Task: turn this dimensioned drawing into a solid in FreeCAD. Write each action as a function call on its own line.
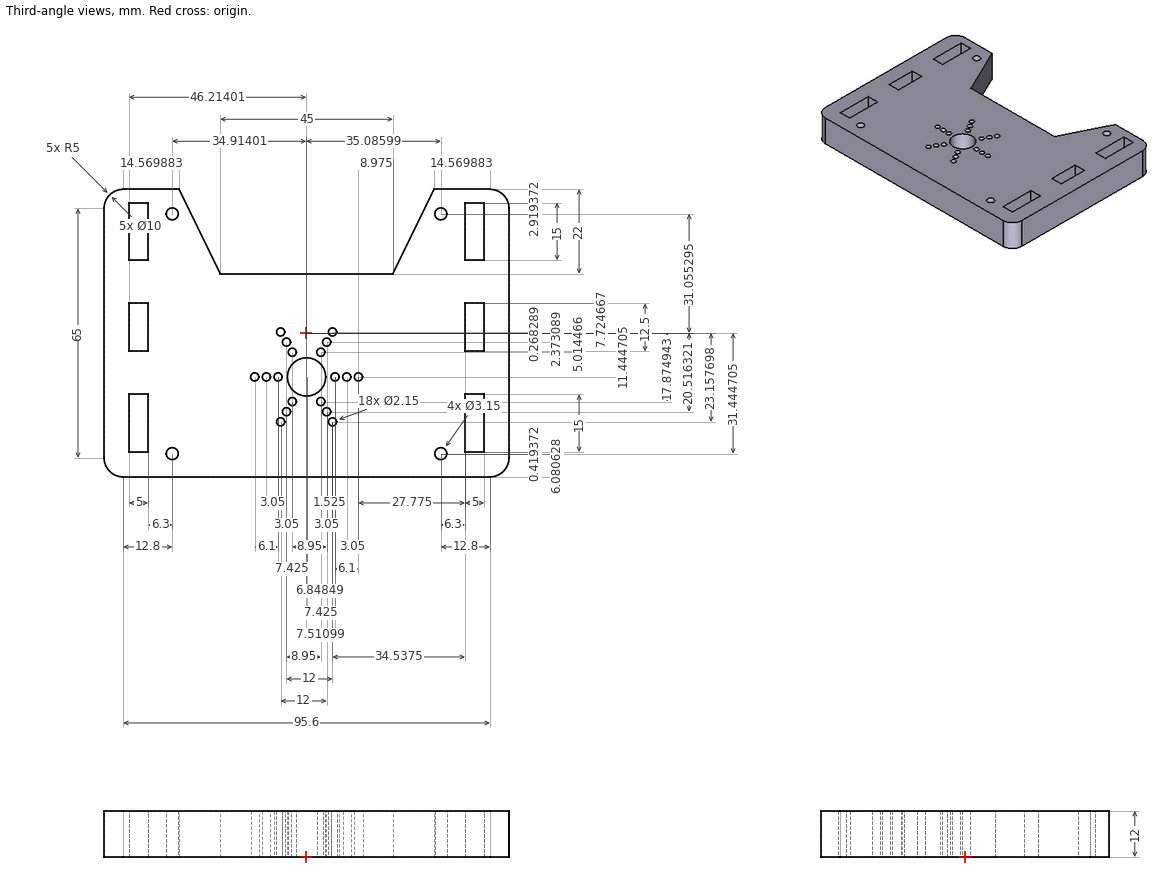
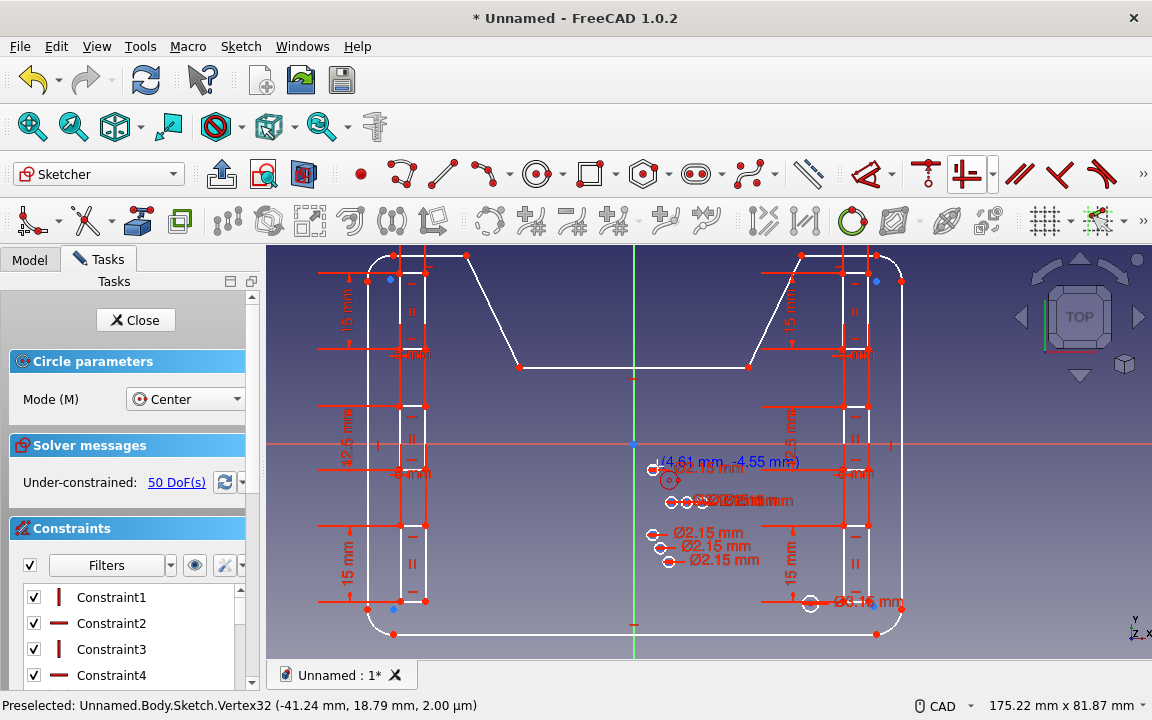
scroll(668, 443, up, 13)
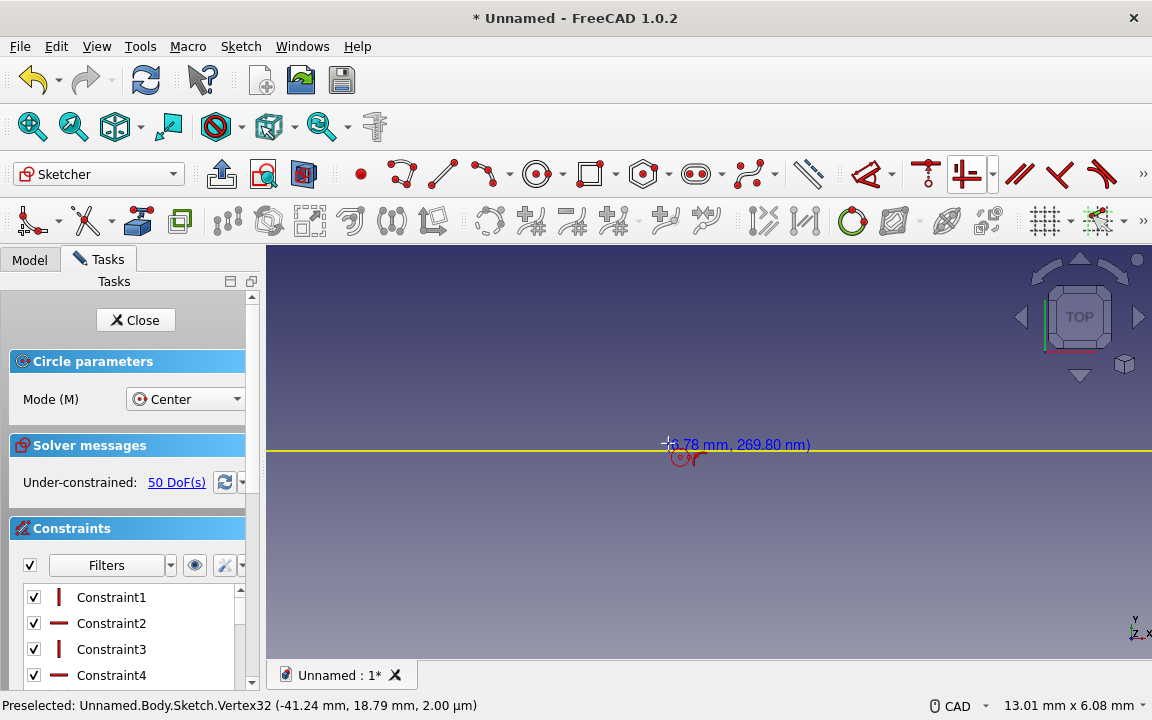
click(667, 432)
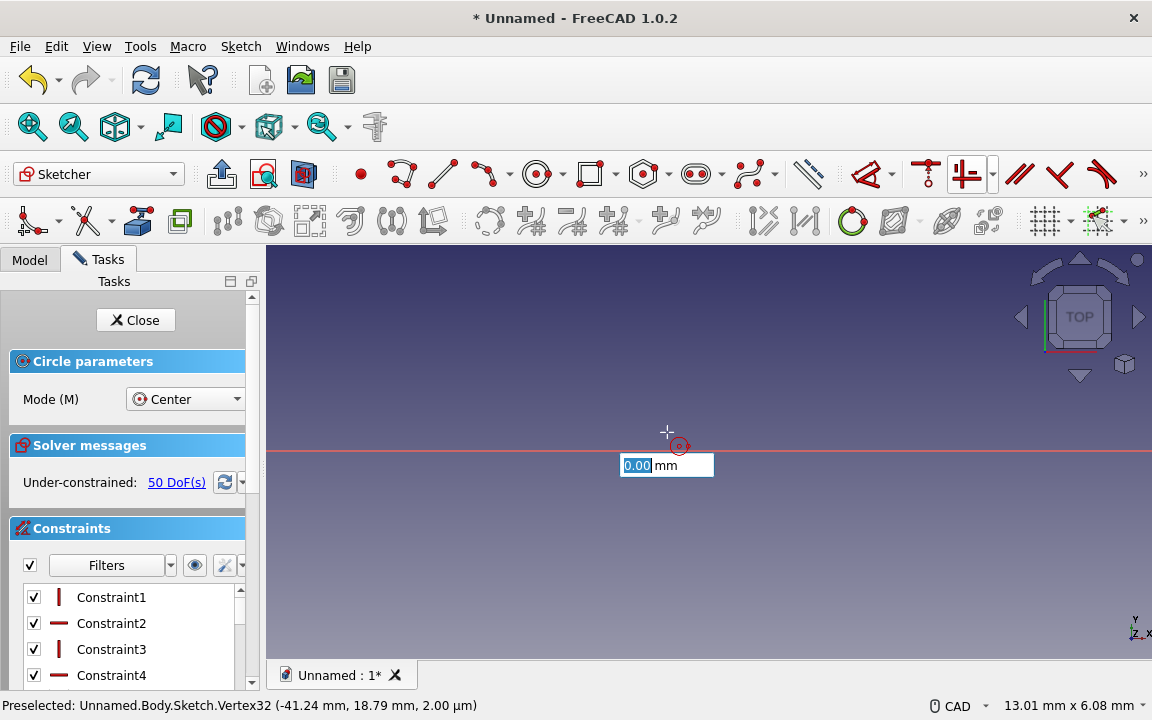
scroll(663, 452, down, 15)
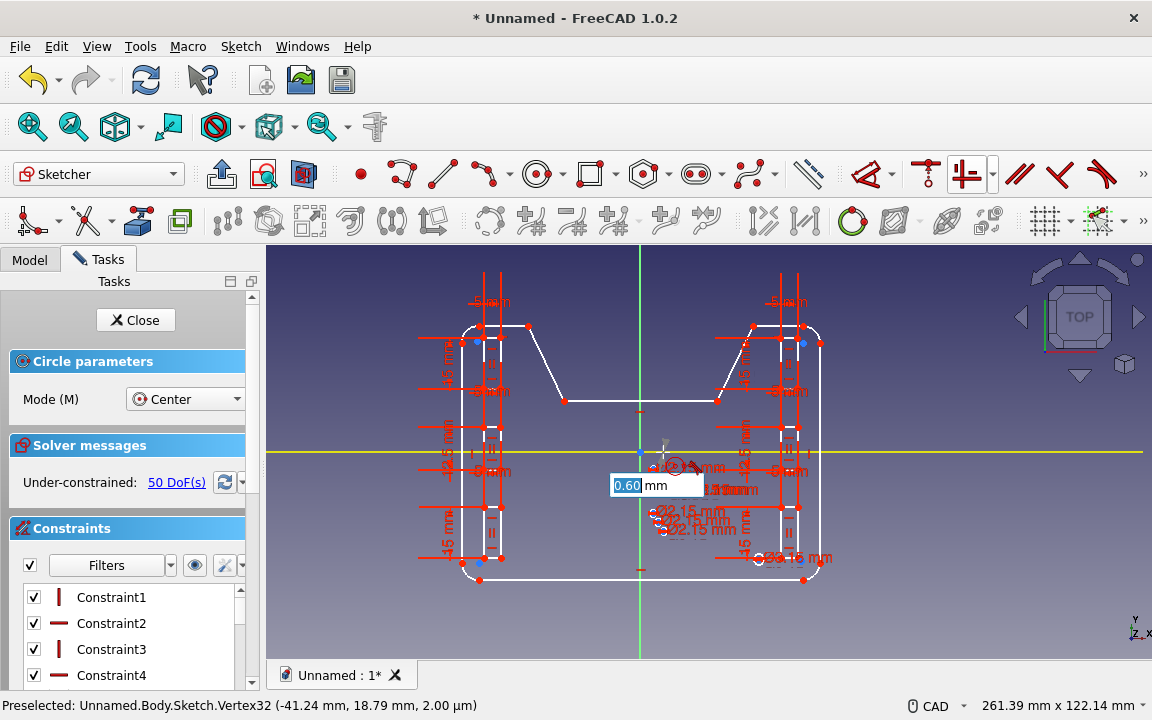
scroll(666, 449, up, 8)
move(665, 447)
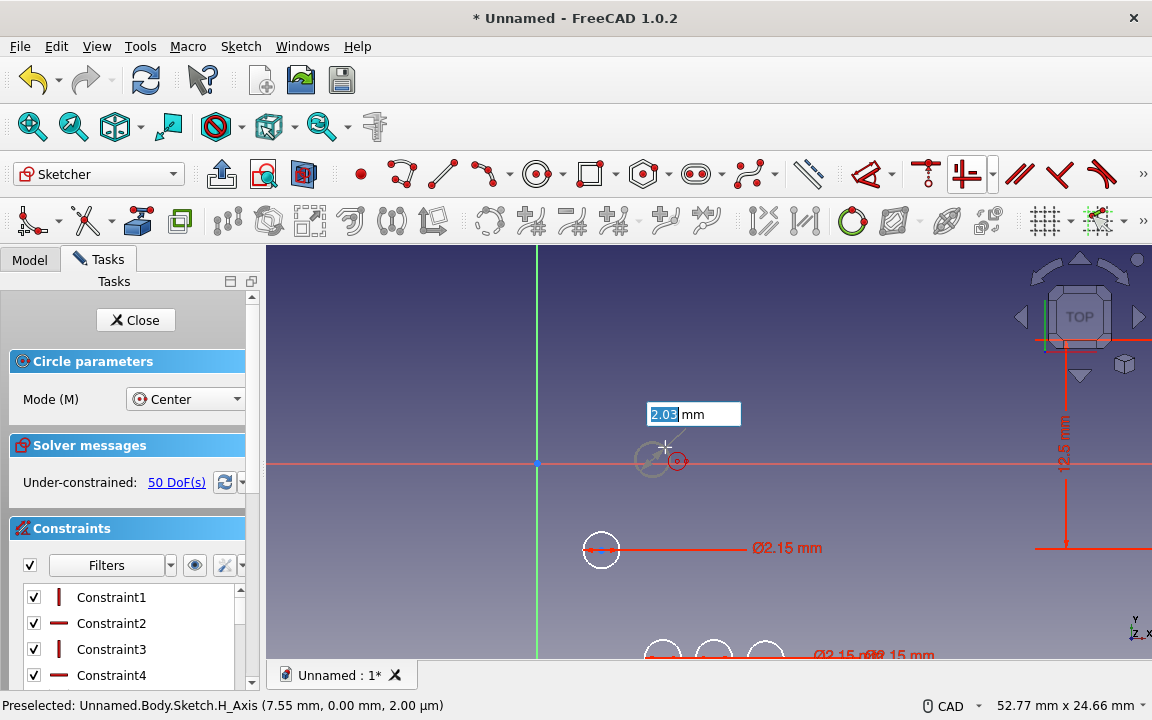
text(2.15)
key(Return)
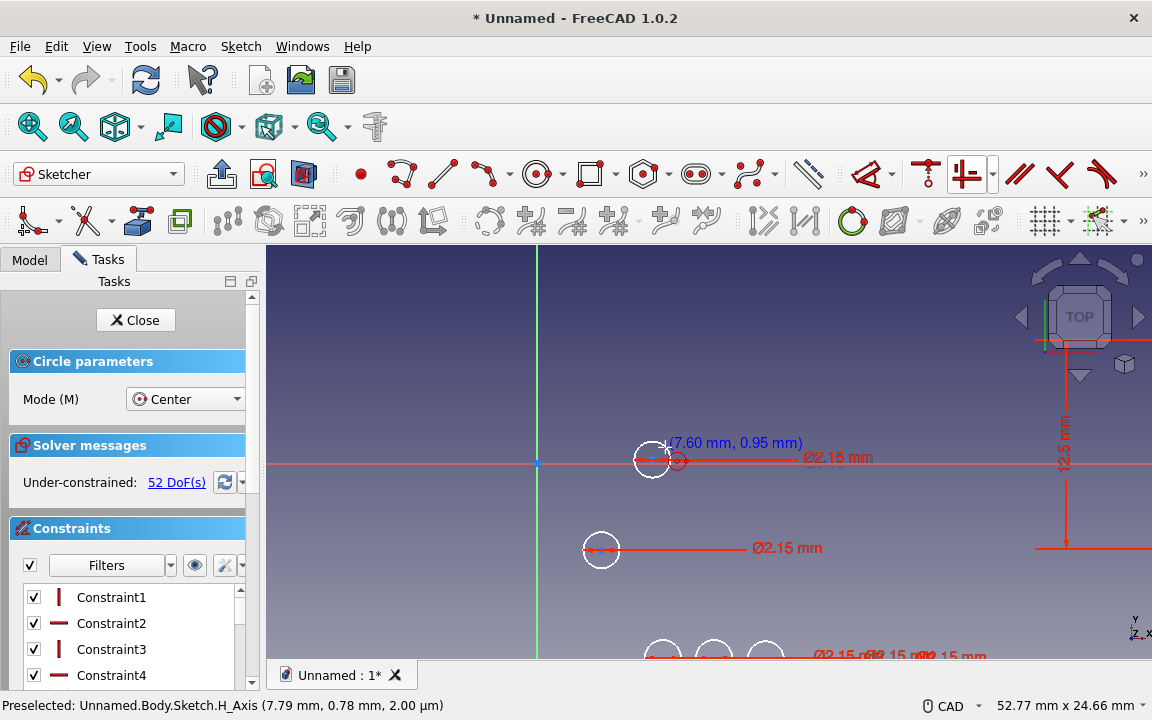
scroll(627, 504, up, 2)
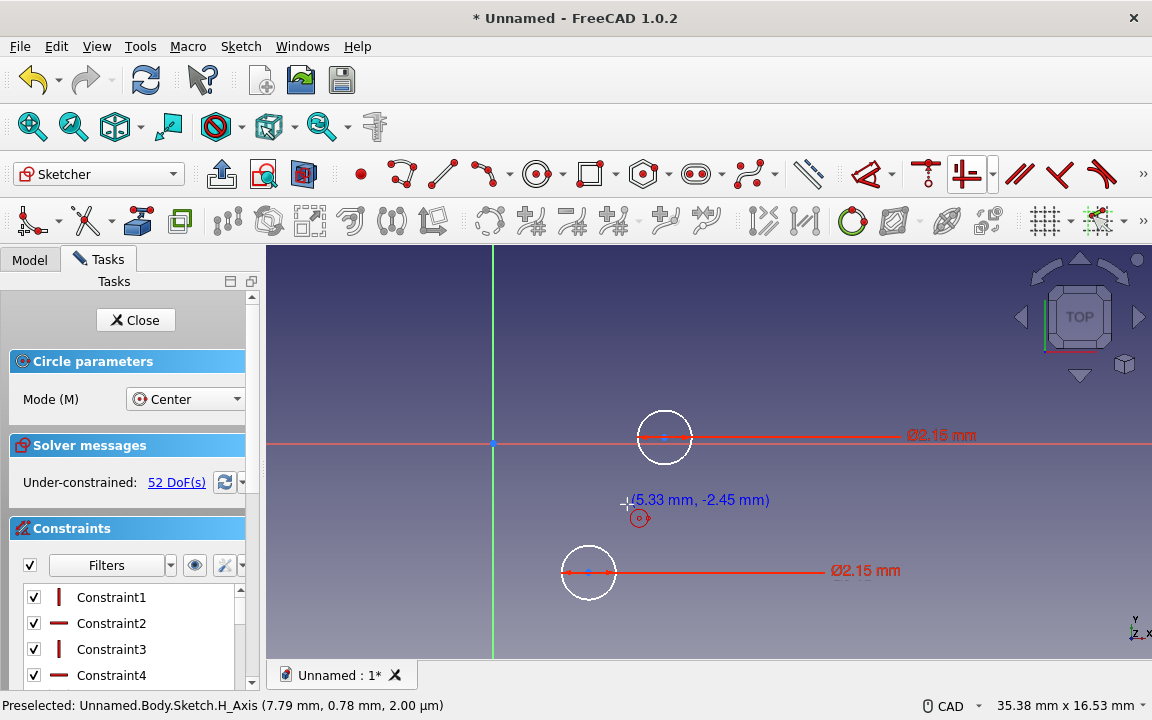
scroll(663, 453, down, 10)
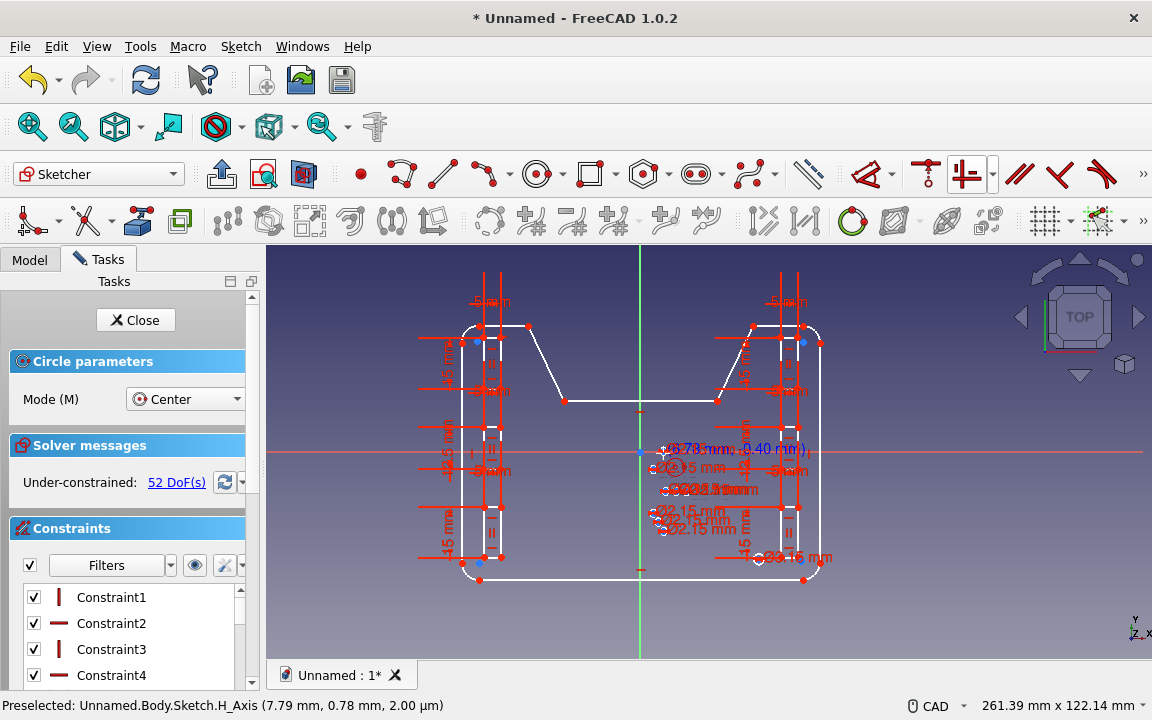
scroll(658, 460, up, 5)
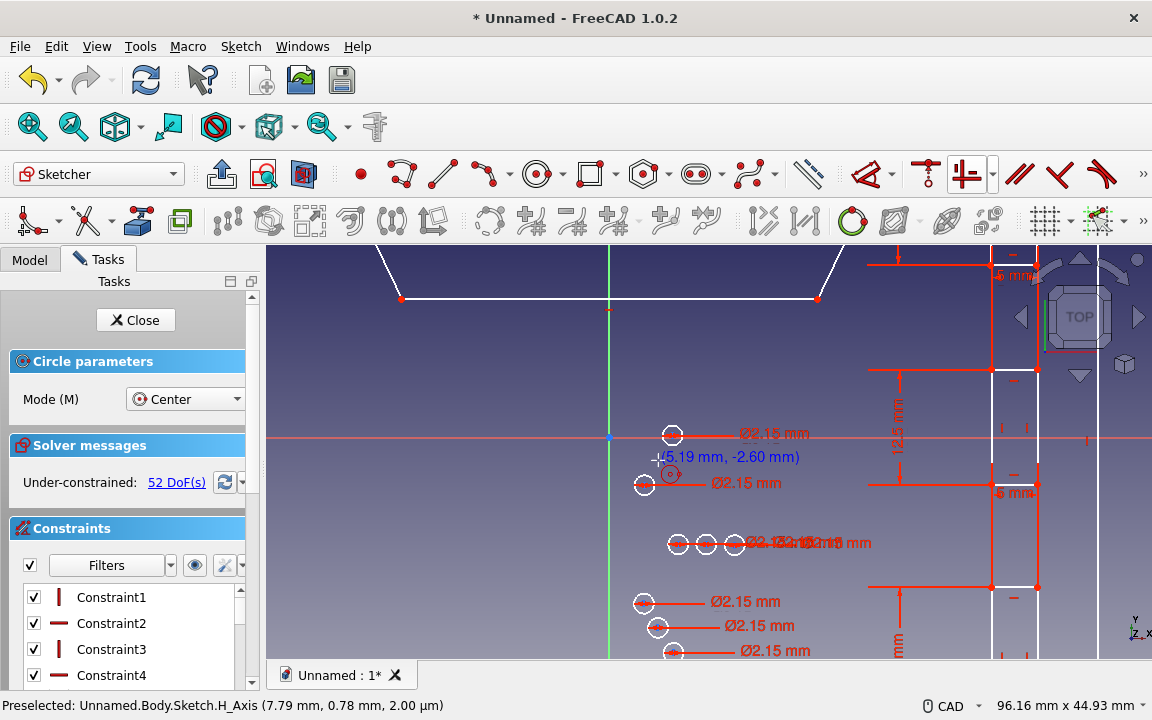
click(658, 460)
move(651, 453)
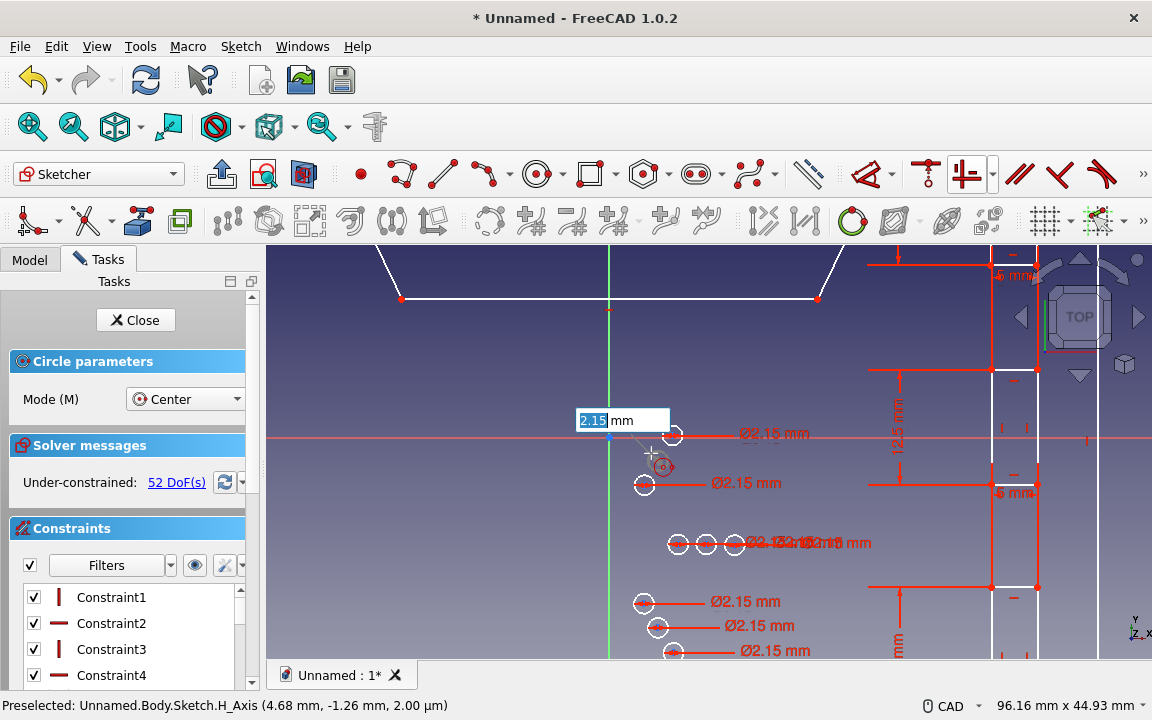
text(2.15)
key(Return)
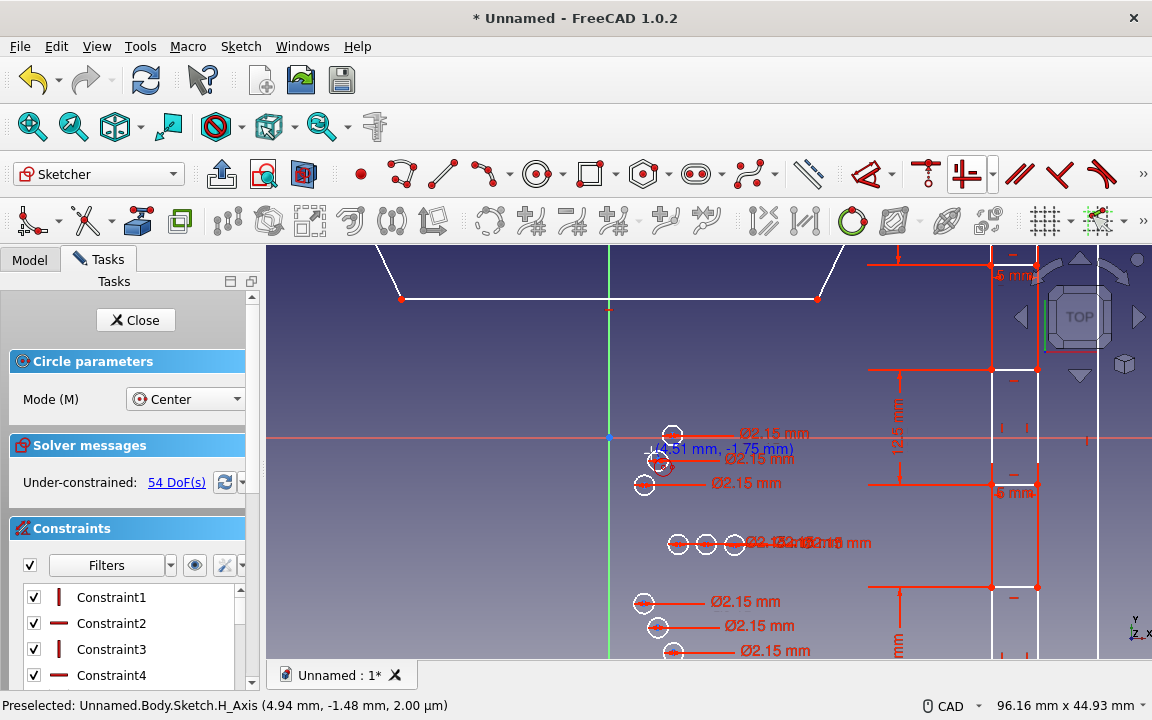
scroll(562, 627, up, 5)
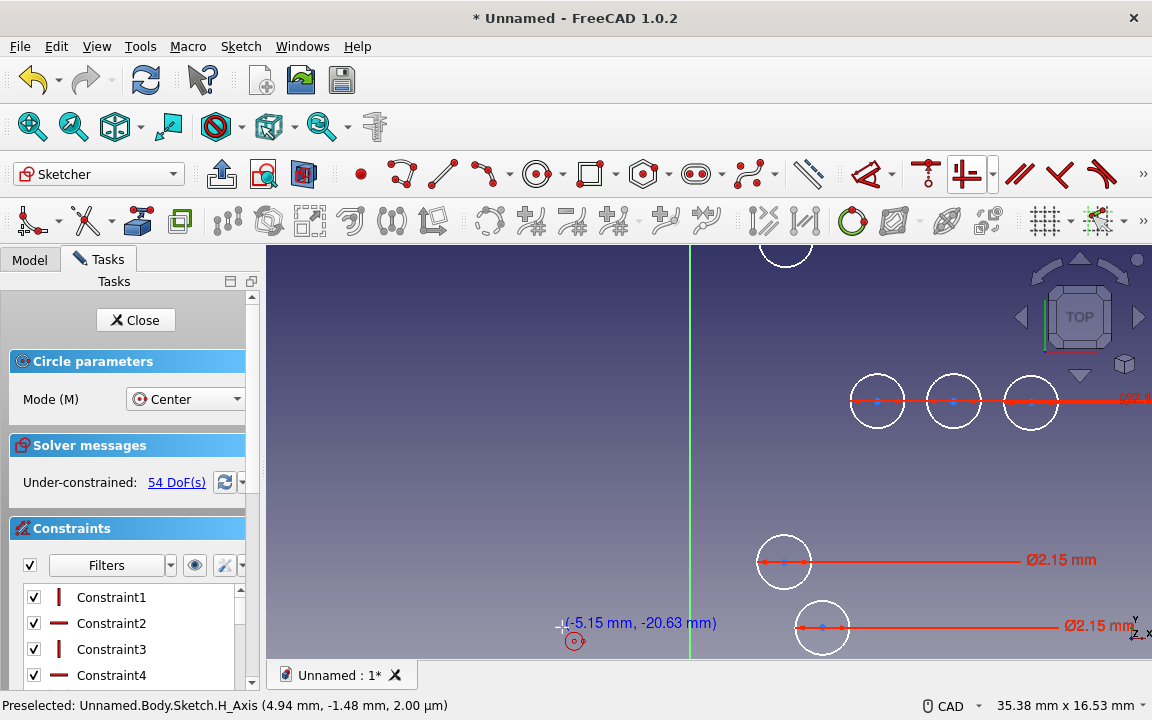
scroll(632, 505, down, 10)